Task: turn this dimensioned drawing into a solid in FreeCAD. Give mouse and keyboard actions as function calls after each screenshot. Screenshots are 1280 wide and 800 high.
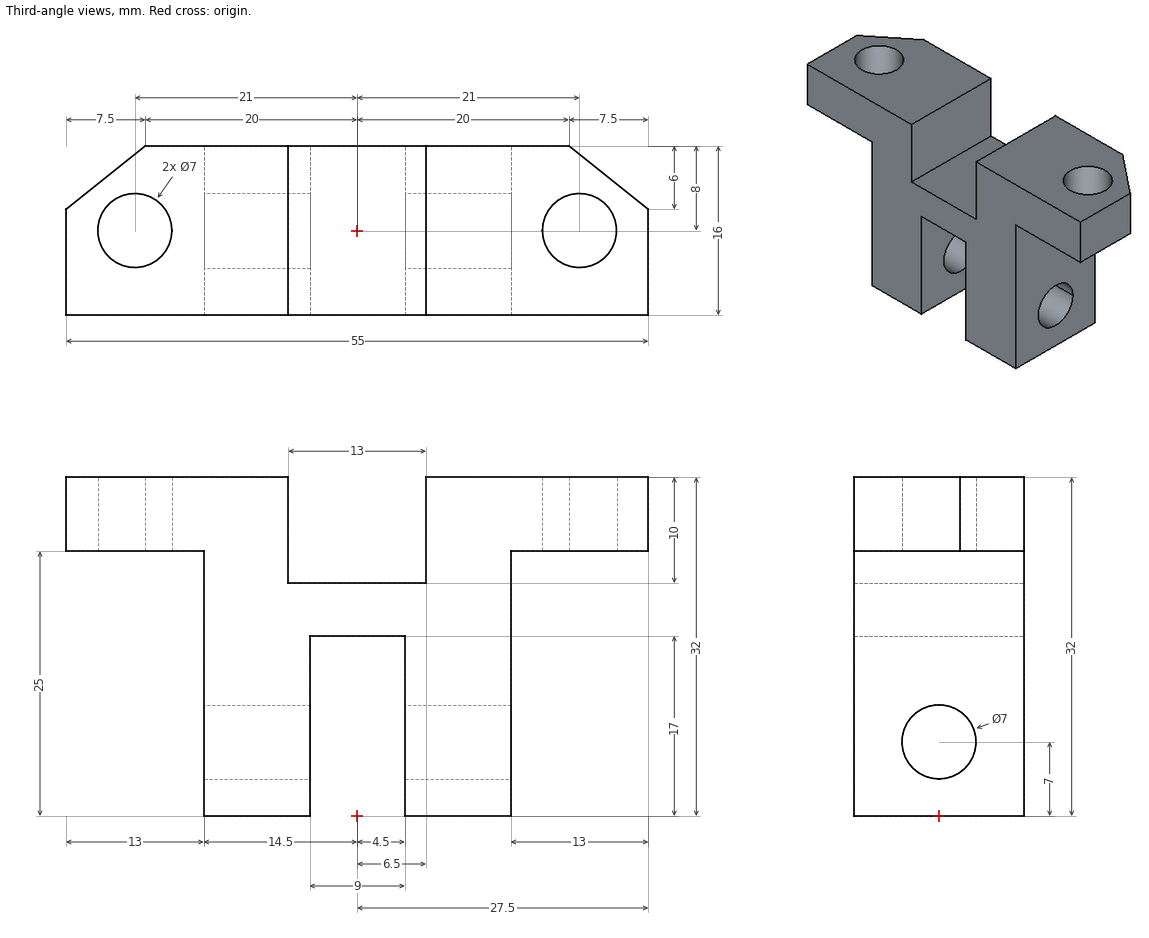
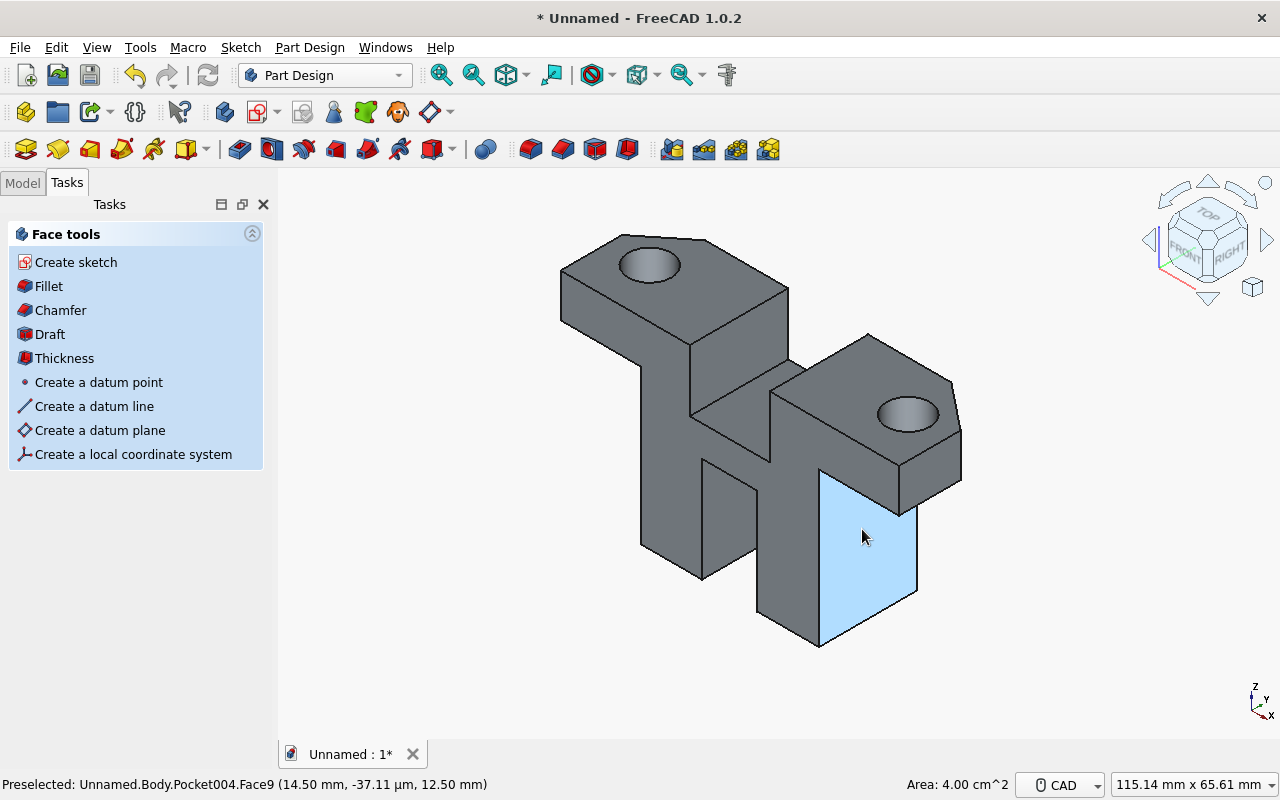
click(258, 112)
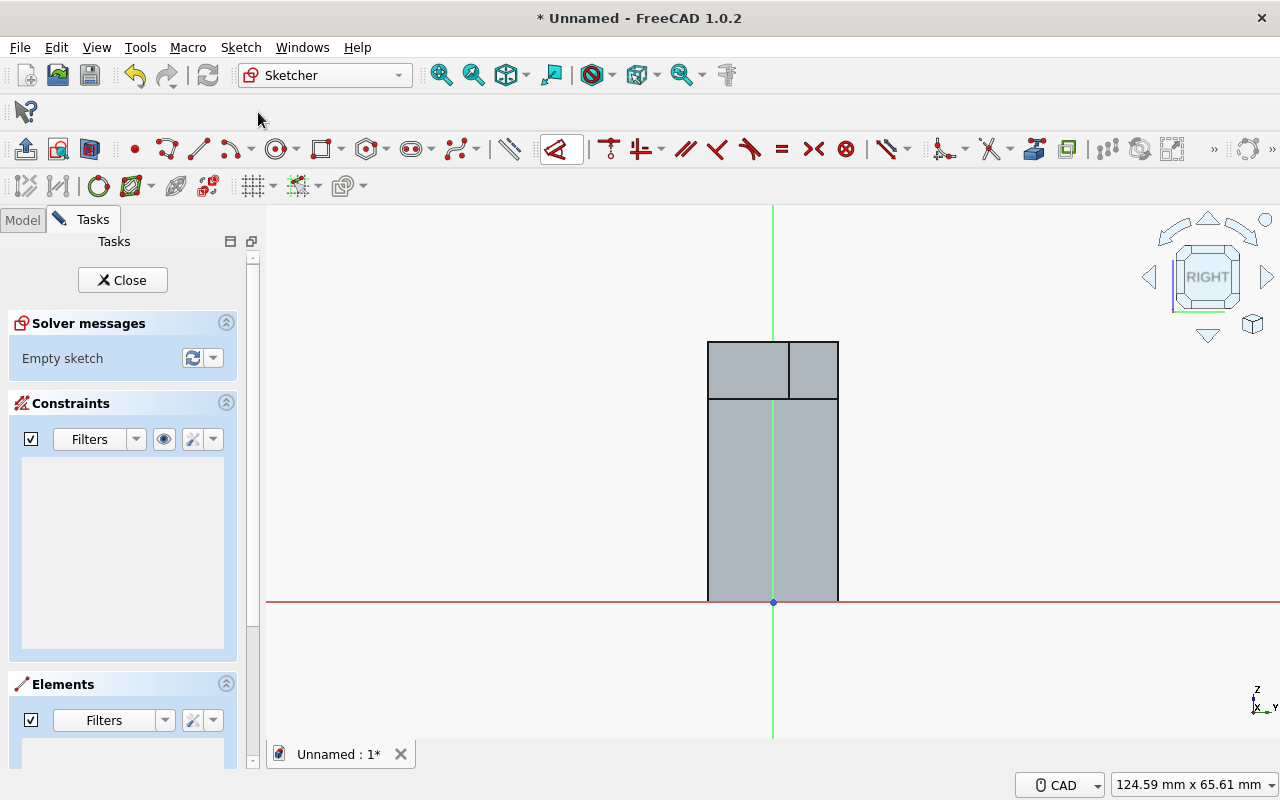
click(90, 150)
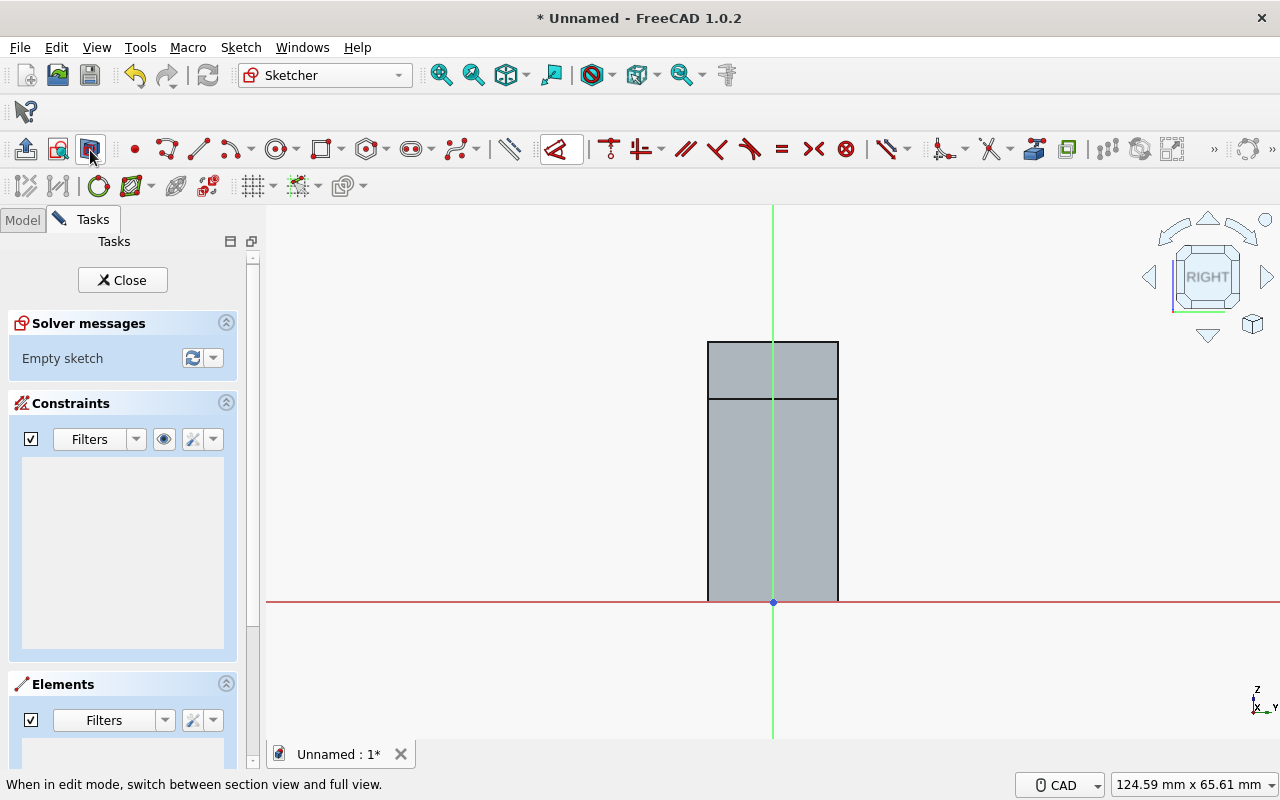
scroll(795, 588, up, 7)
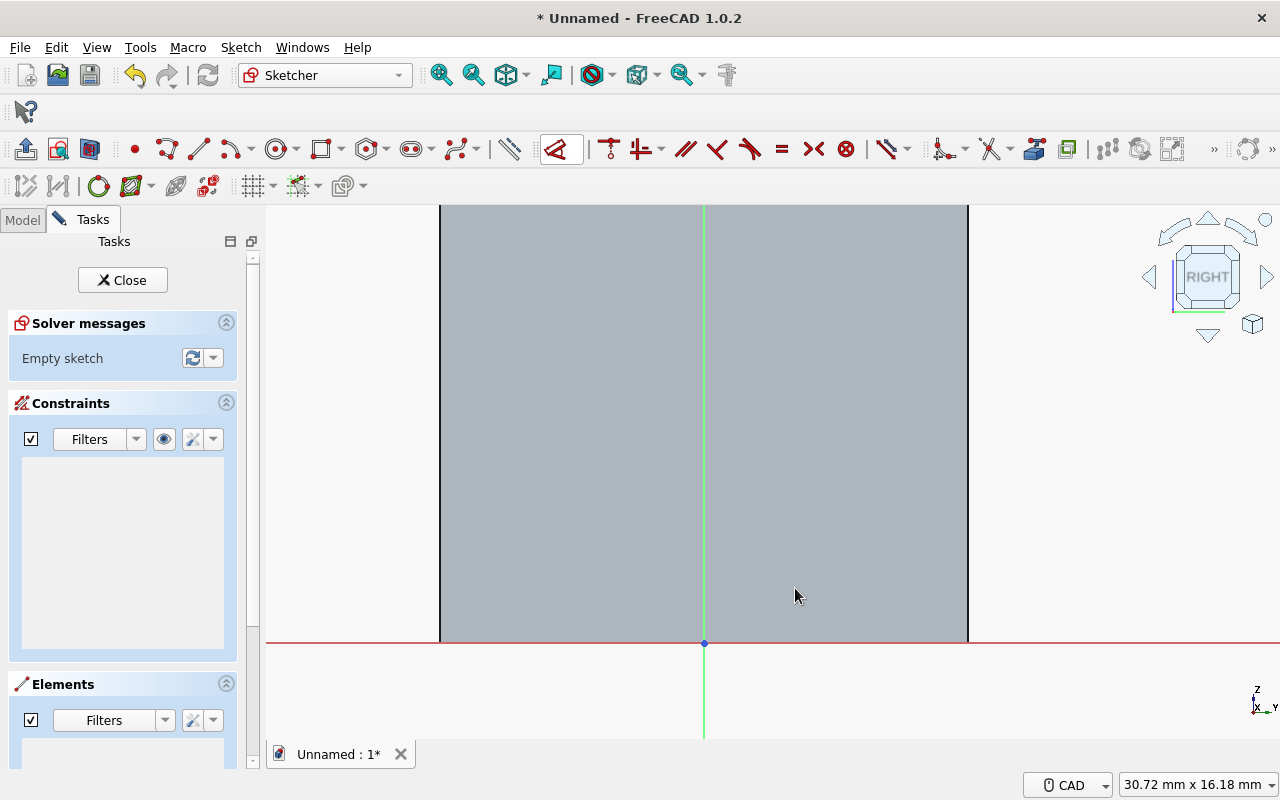
click(276, 150)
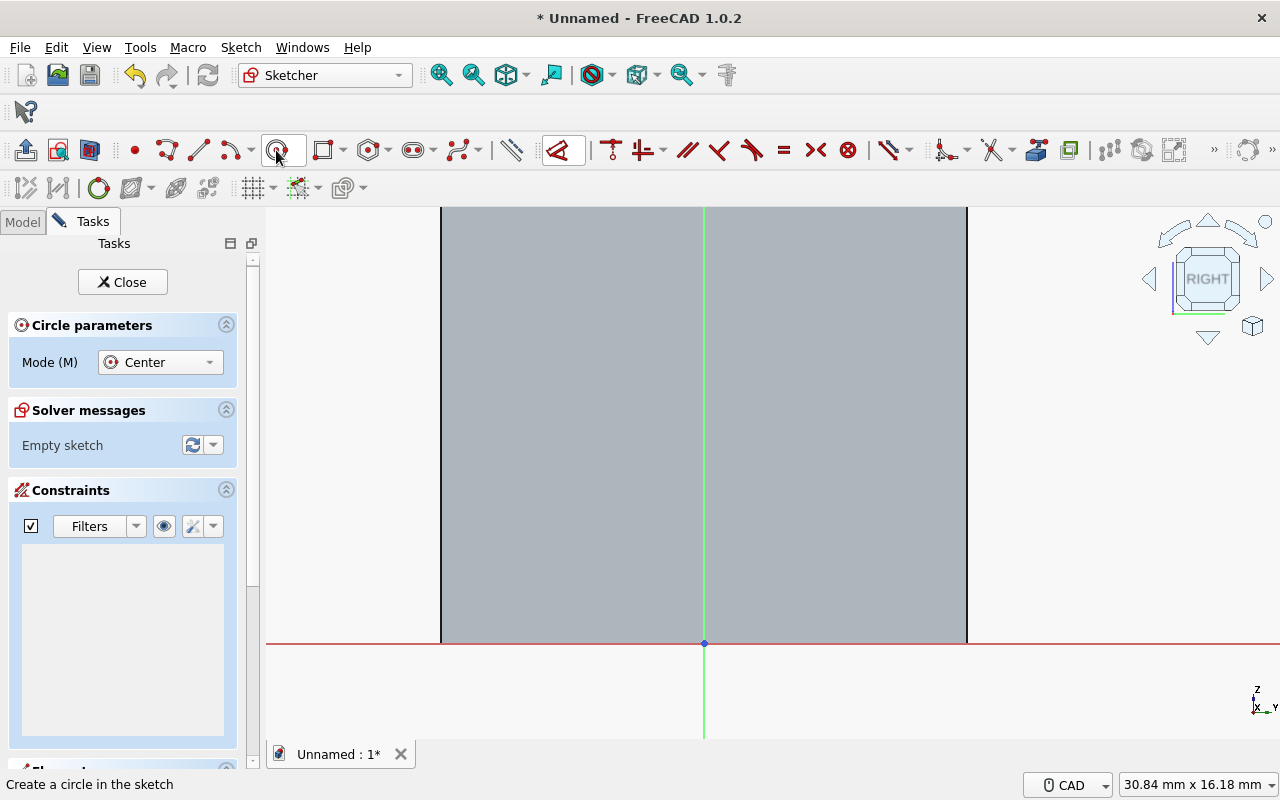
click(704, 414)
click(786, 332)
key(Escape)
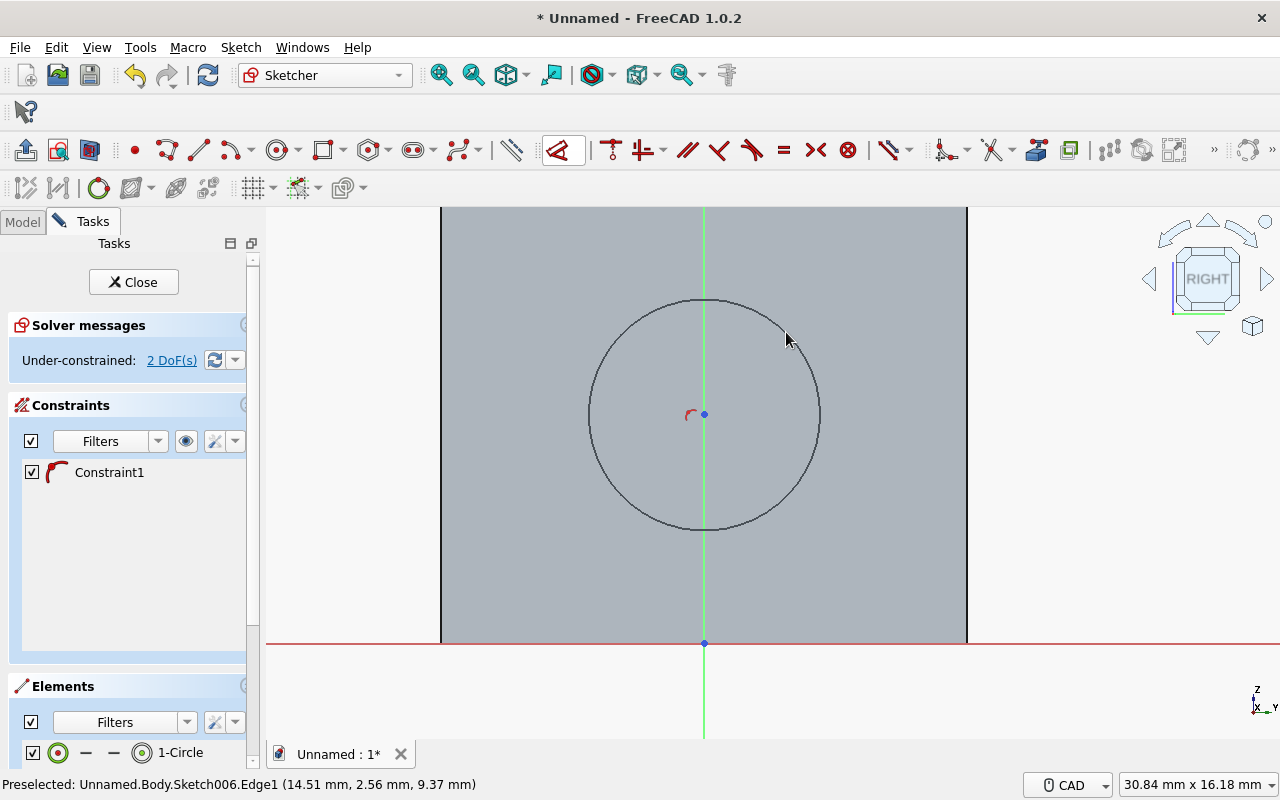
click(786, 333)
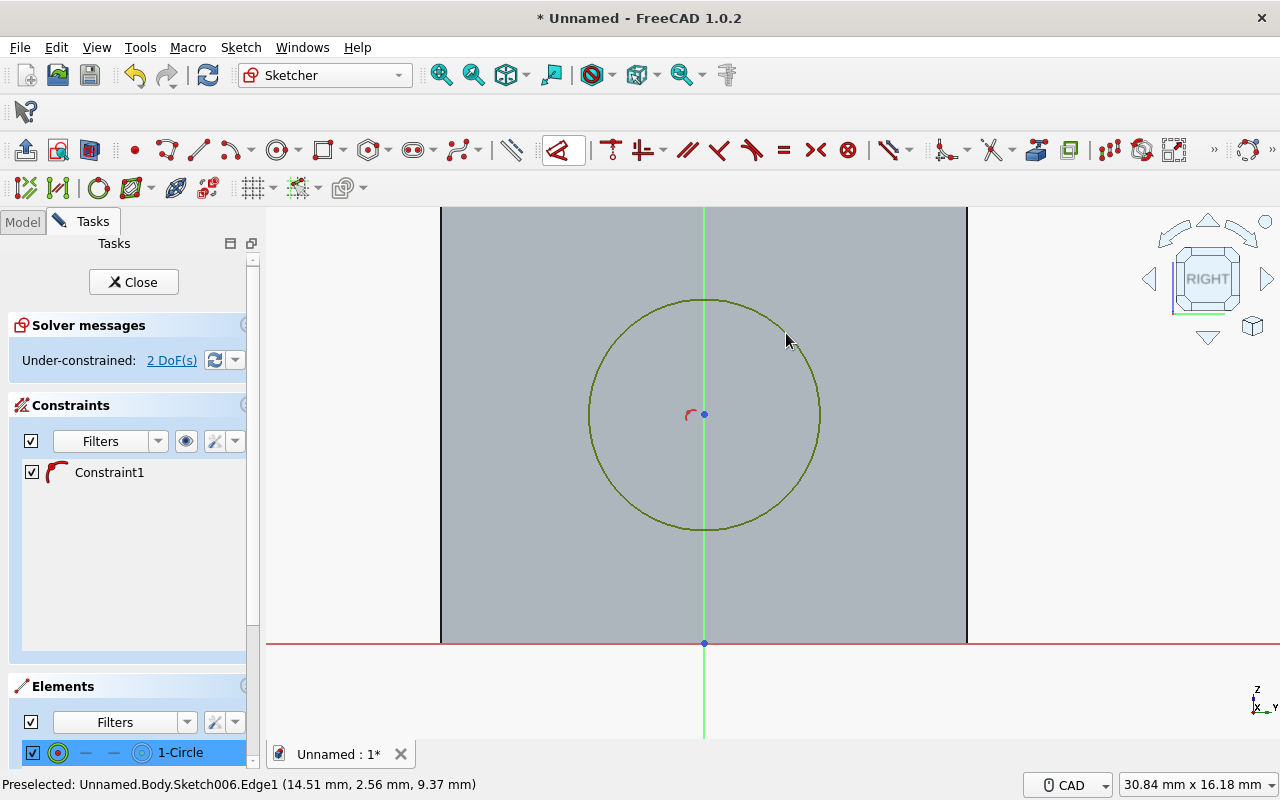
key(k)
key(o)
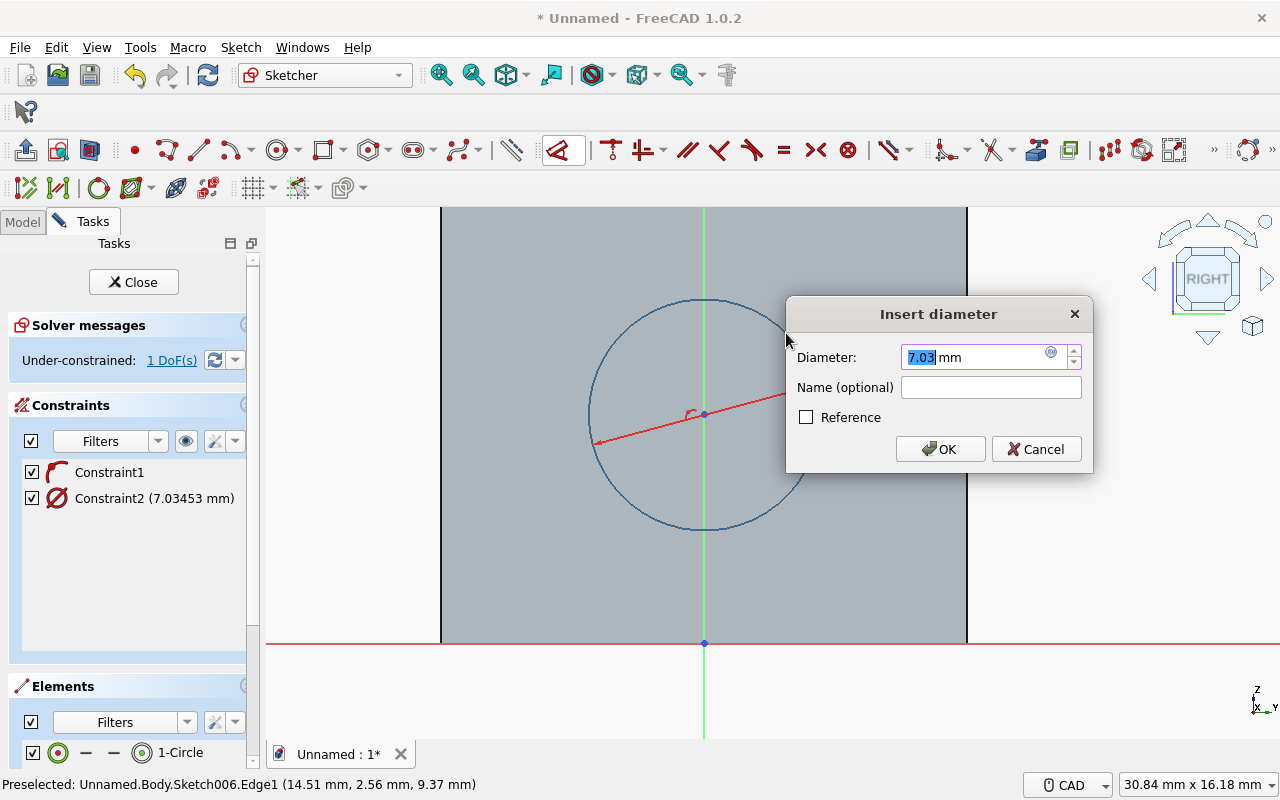
text(7)
key(Return)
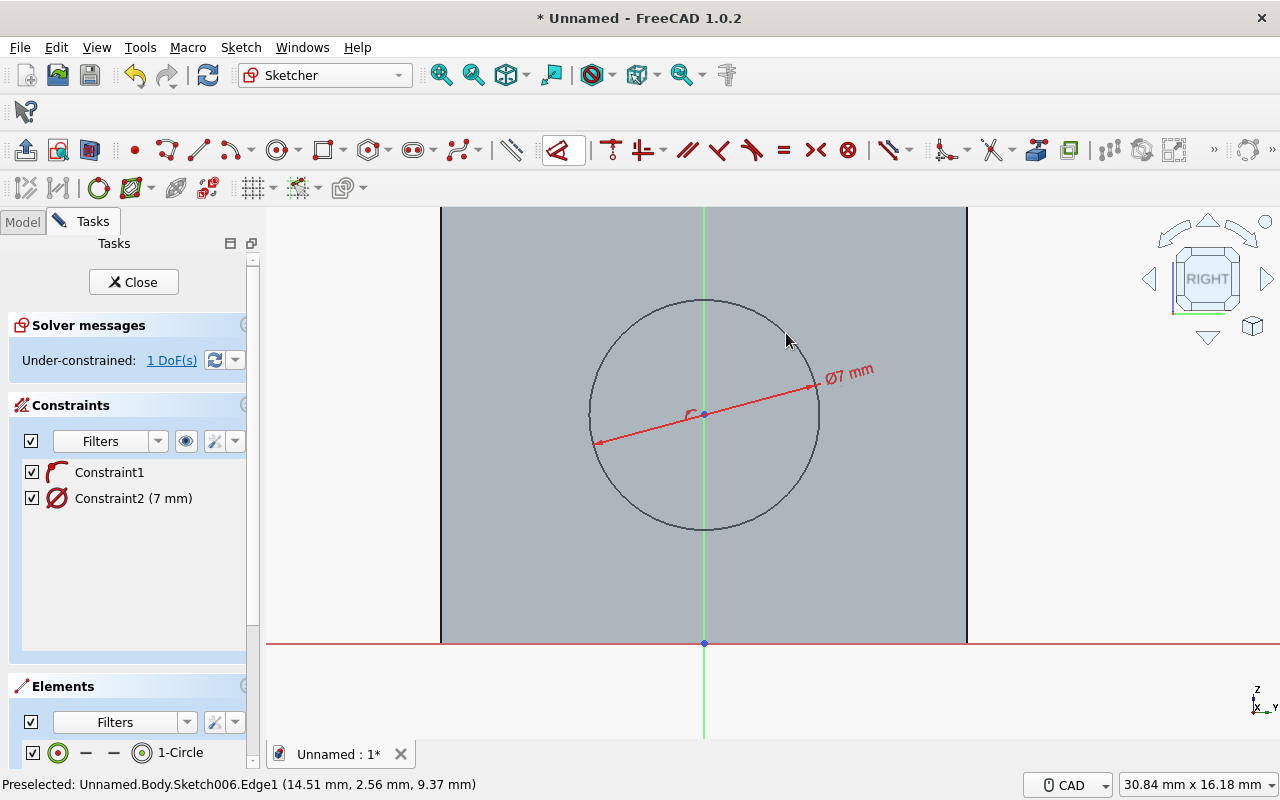
click(704, 415)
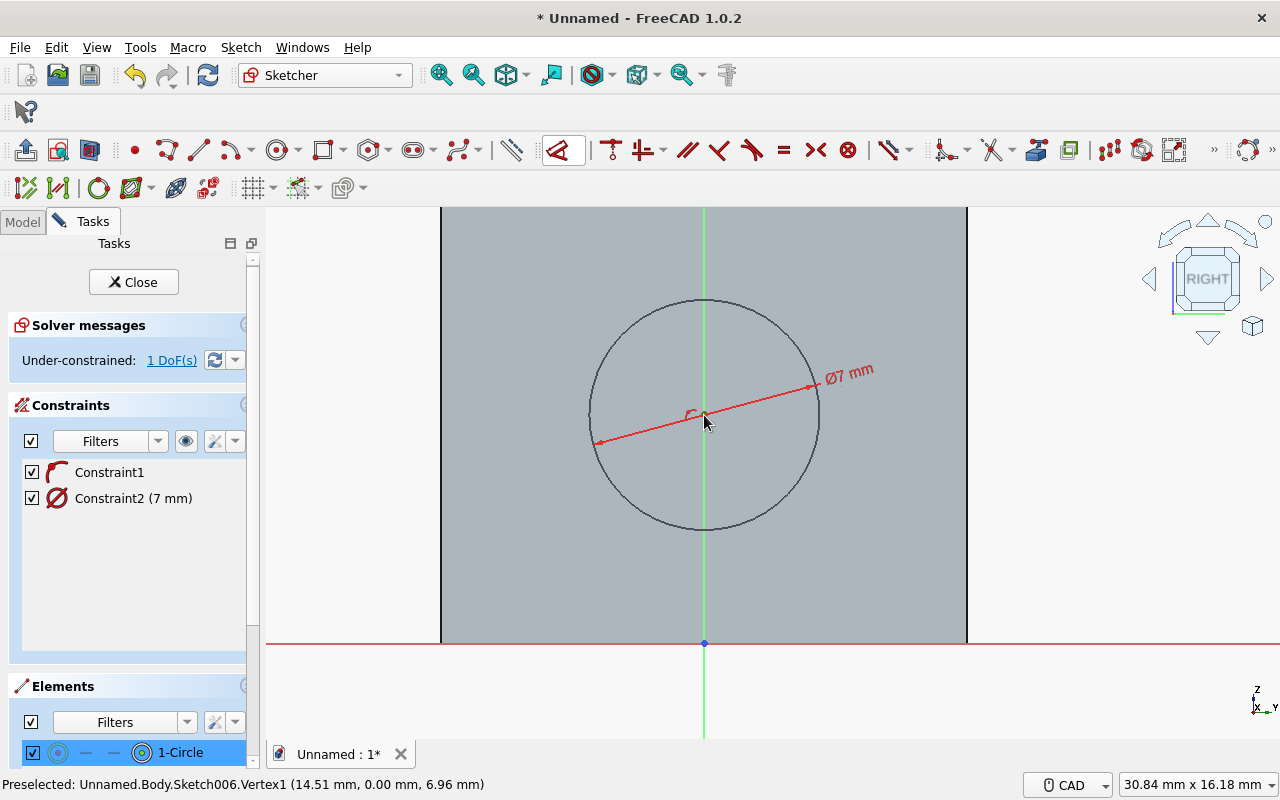
click(580, 150)